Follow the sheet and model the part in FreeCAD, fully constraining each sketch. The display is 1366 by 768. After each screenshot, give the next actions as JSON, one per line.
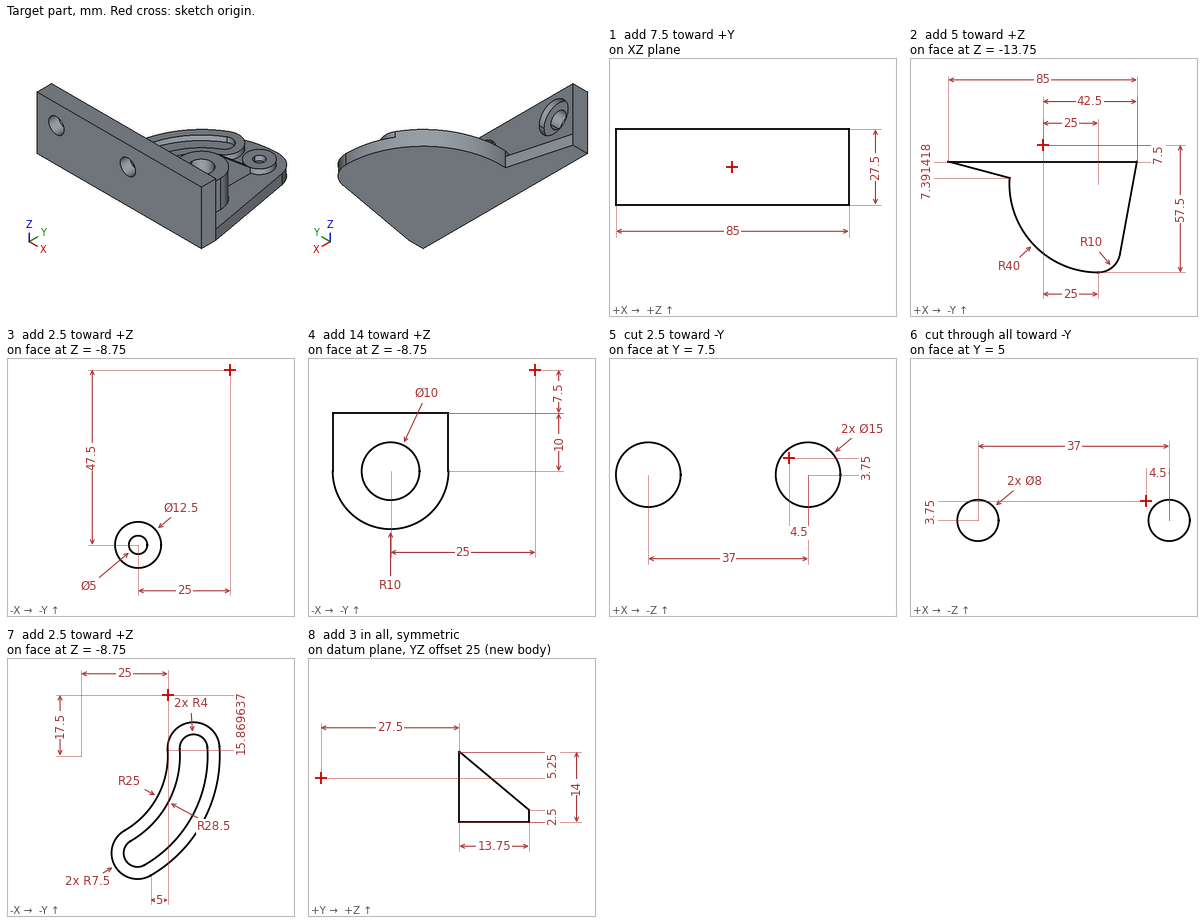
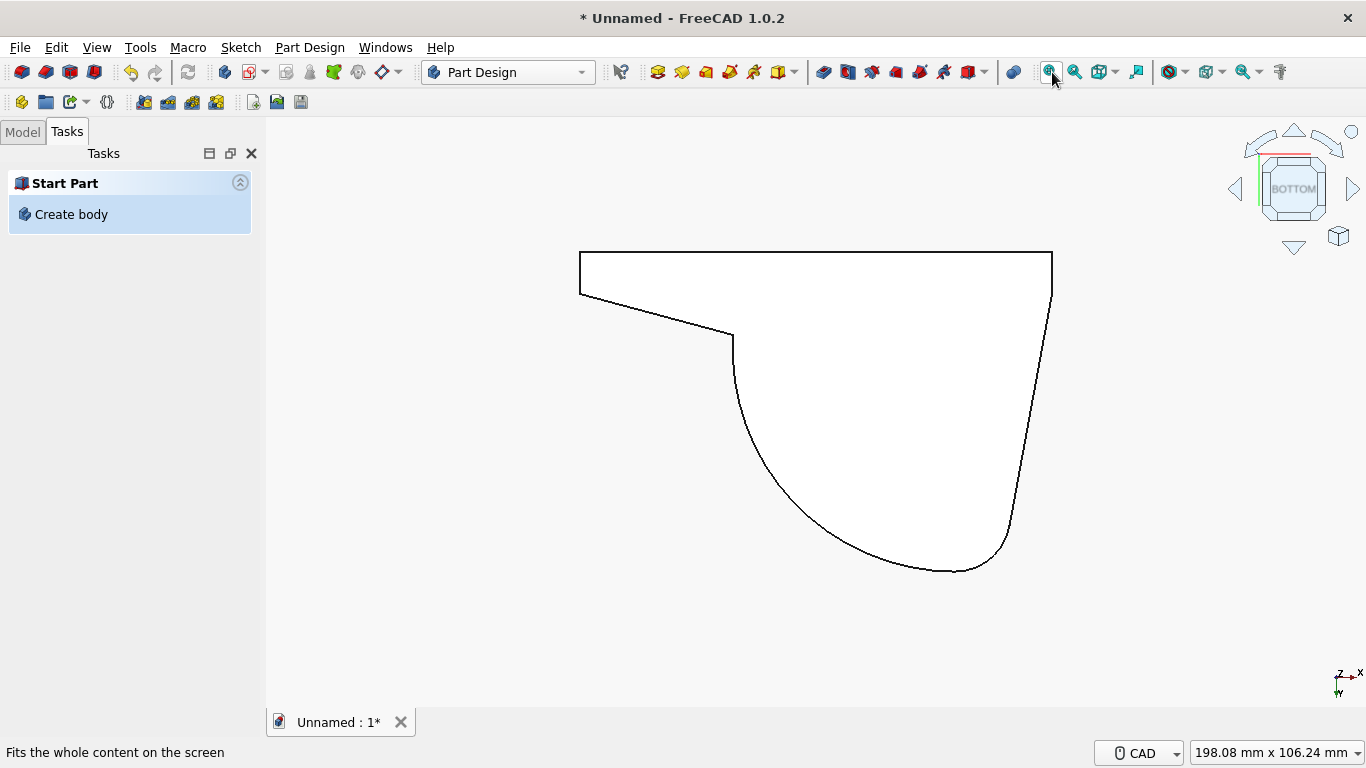
{"action": "key", "text": "0"}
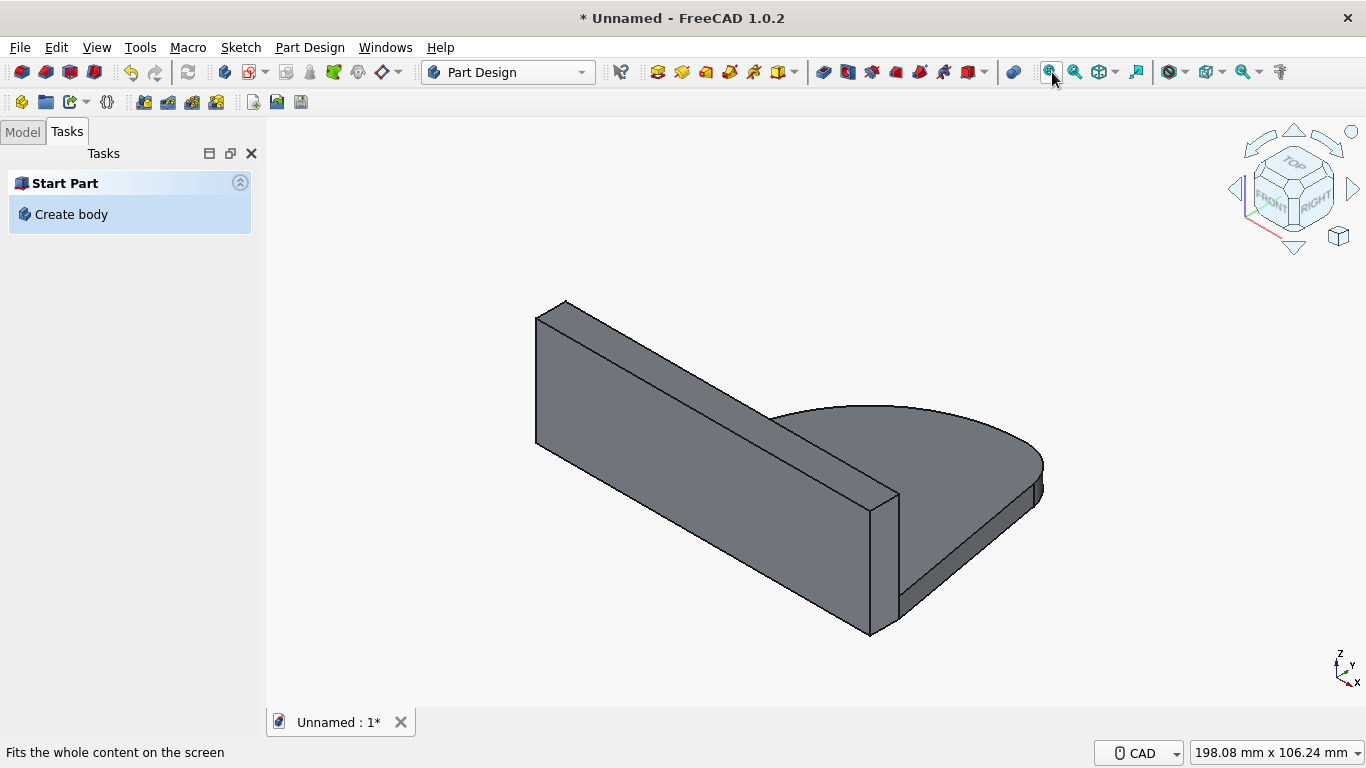
{"action": "left_click", "coordinate": [878, 470]}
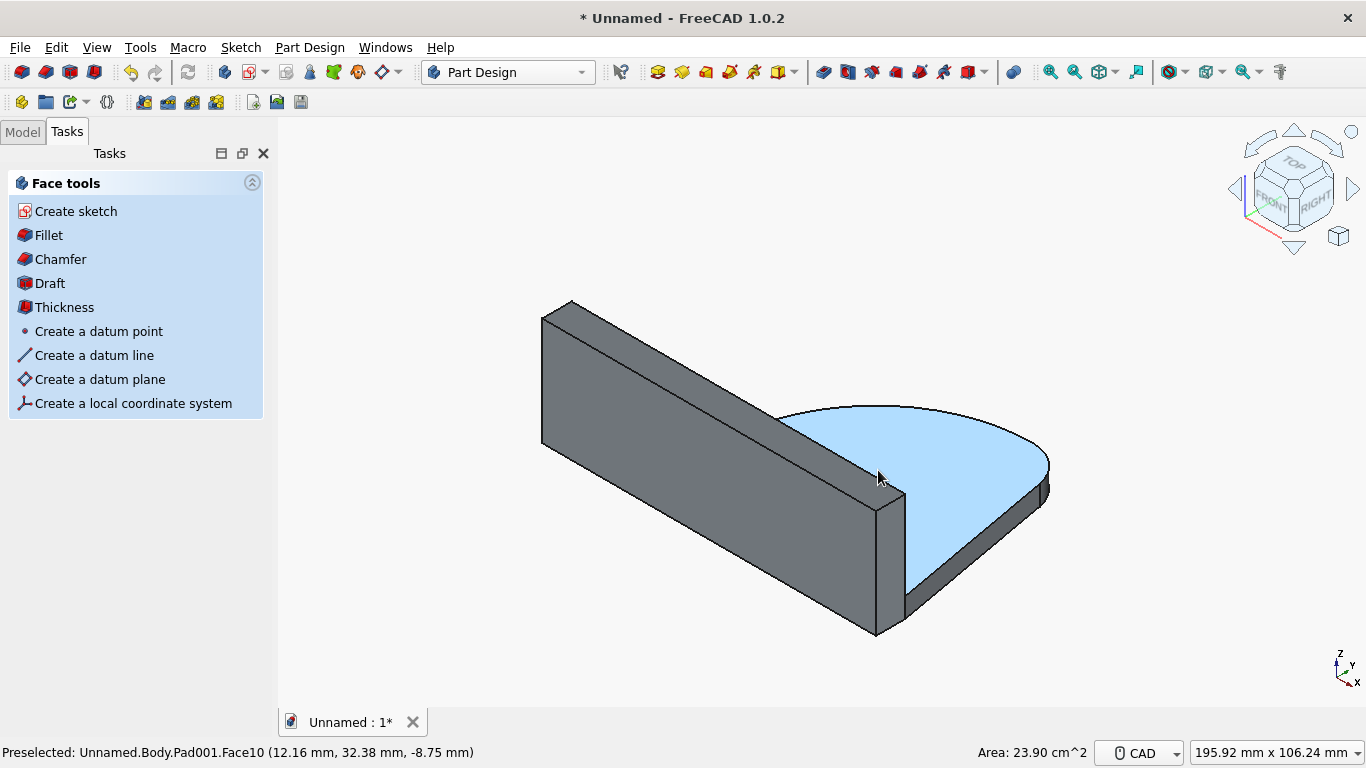
{"action": "left_click", "coordinate": [250, 72]}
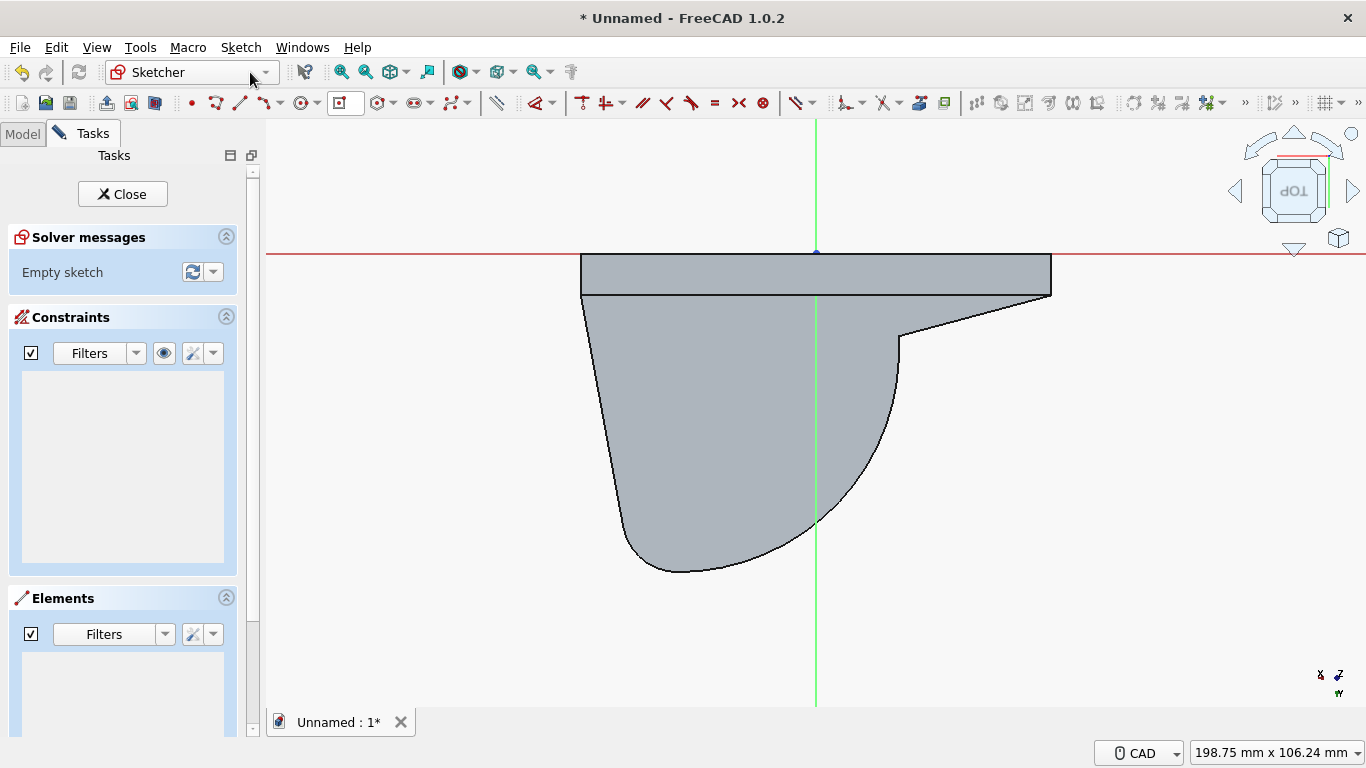
{"action": "left_click", "coordinate": [156, 104]}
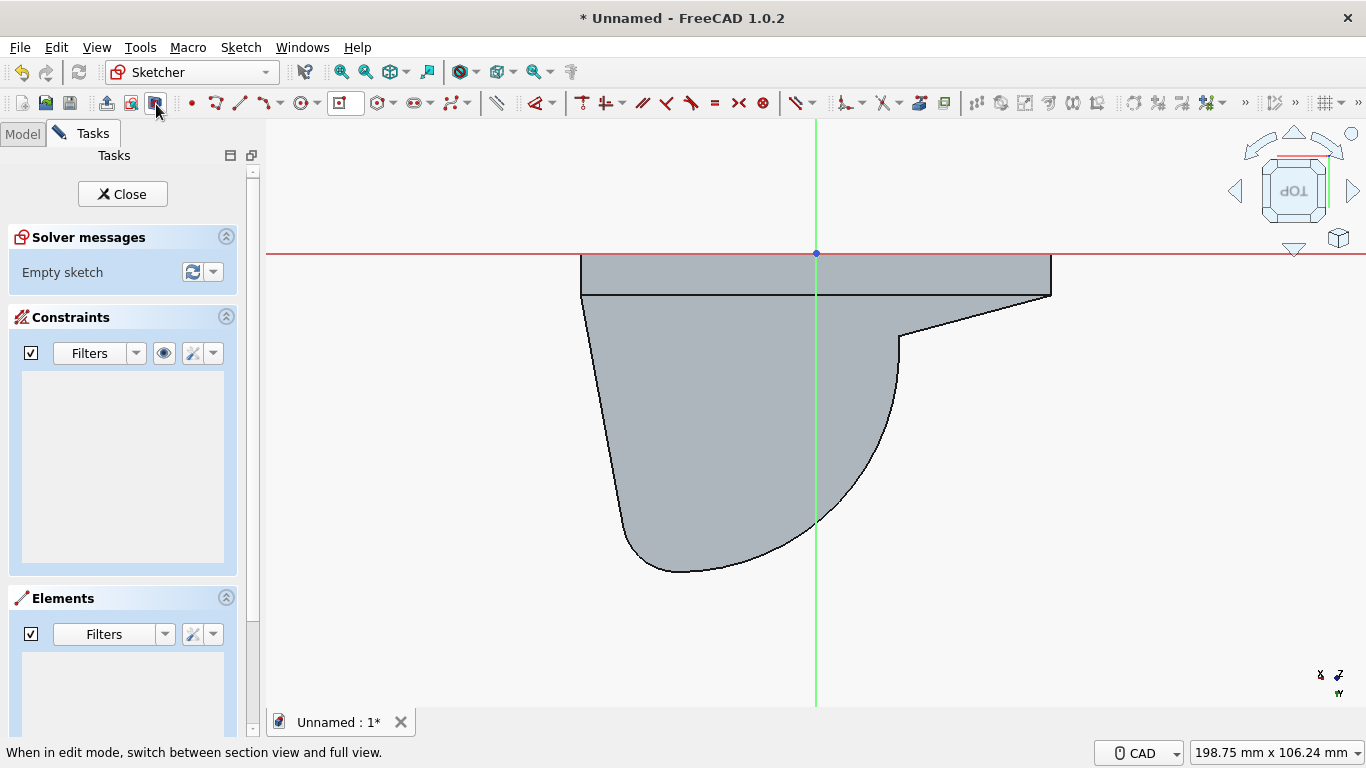
{"action": "scroll", "coordinate": [660, 543], "scroll_direction": "up", "scroll_amount": 8}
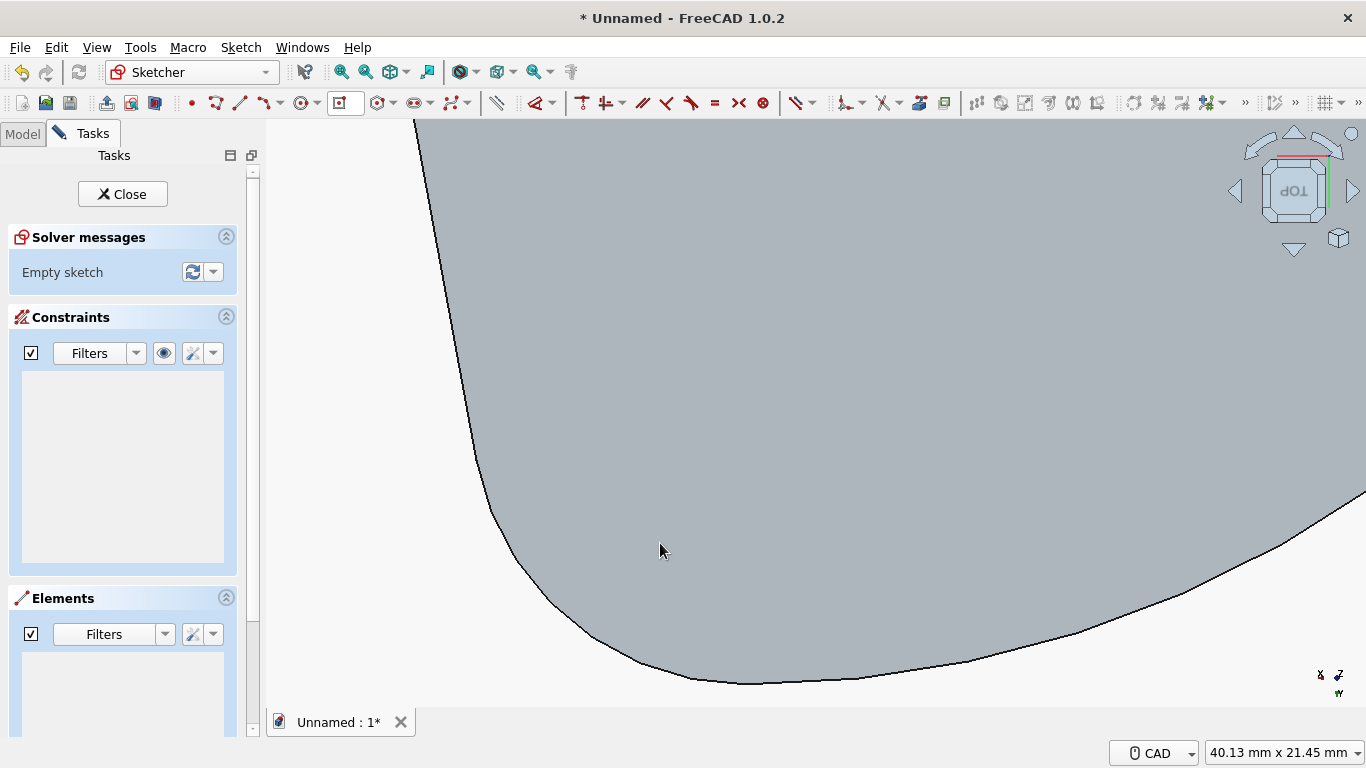
{"action": "left_click", "coordinate": [302, 104]}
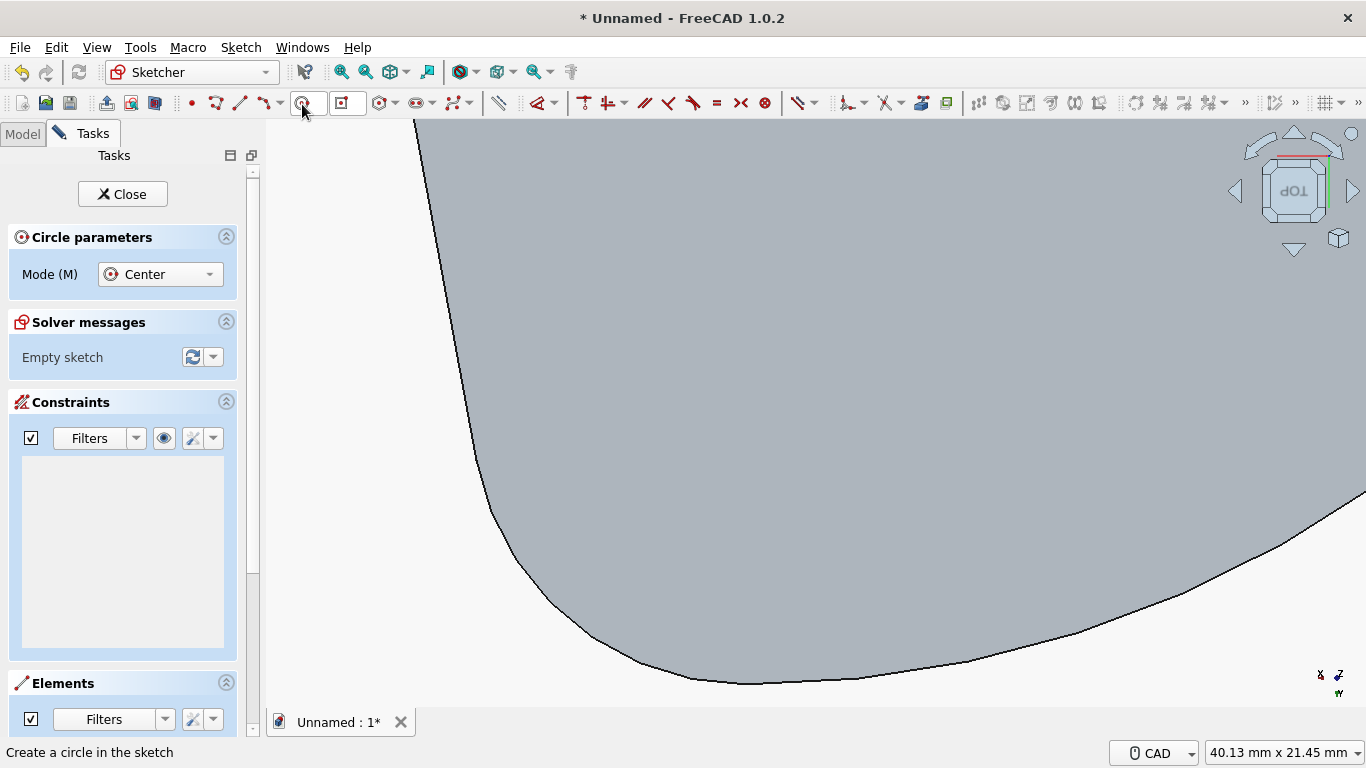
{"action": "left_click", "coordinate": [746, 410]}
{"action": "mouse_move", "coordinate": [867, 289]}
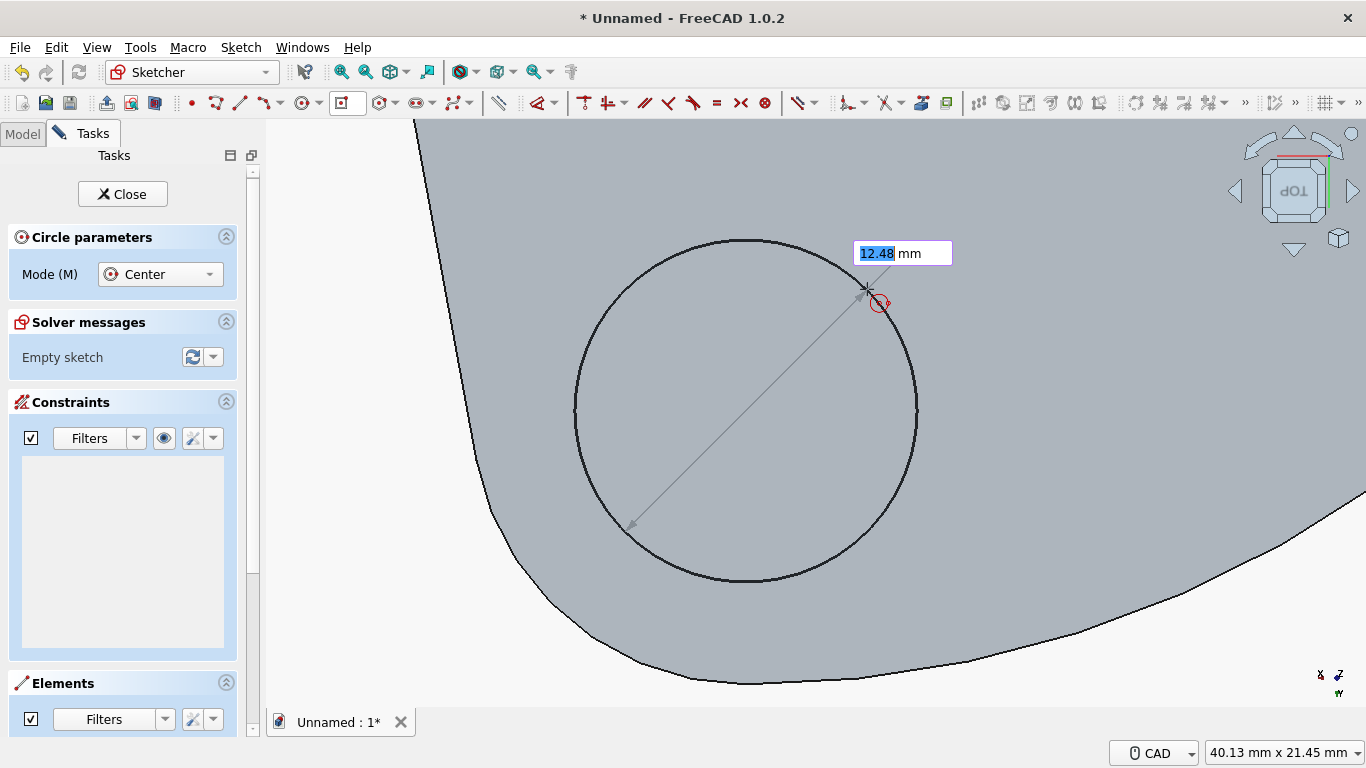
{"action": "type", "text": "12.5"}
{"action": "key", "text": "Return"}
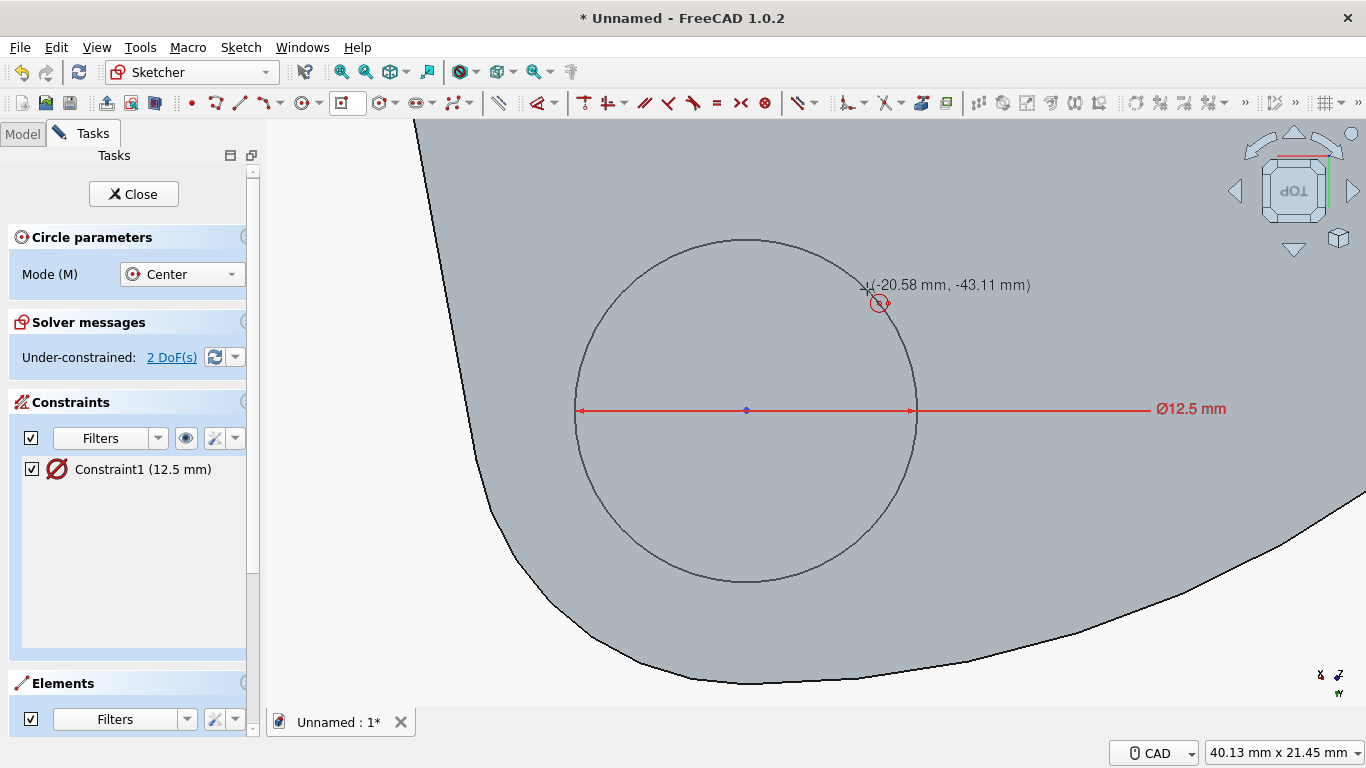
{"action": "left_click", "coordinate": [746, 411]}
{"action": "mouse_move", "coordinate": [794, 362]}